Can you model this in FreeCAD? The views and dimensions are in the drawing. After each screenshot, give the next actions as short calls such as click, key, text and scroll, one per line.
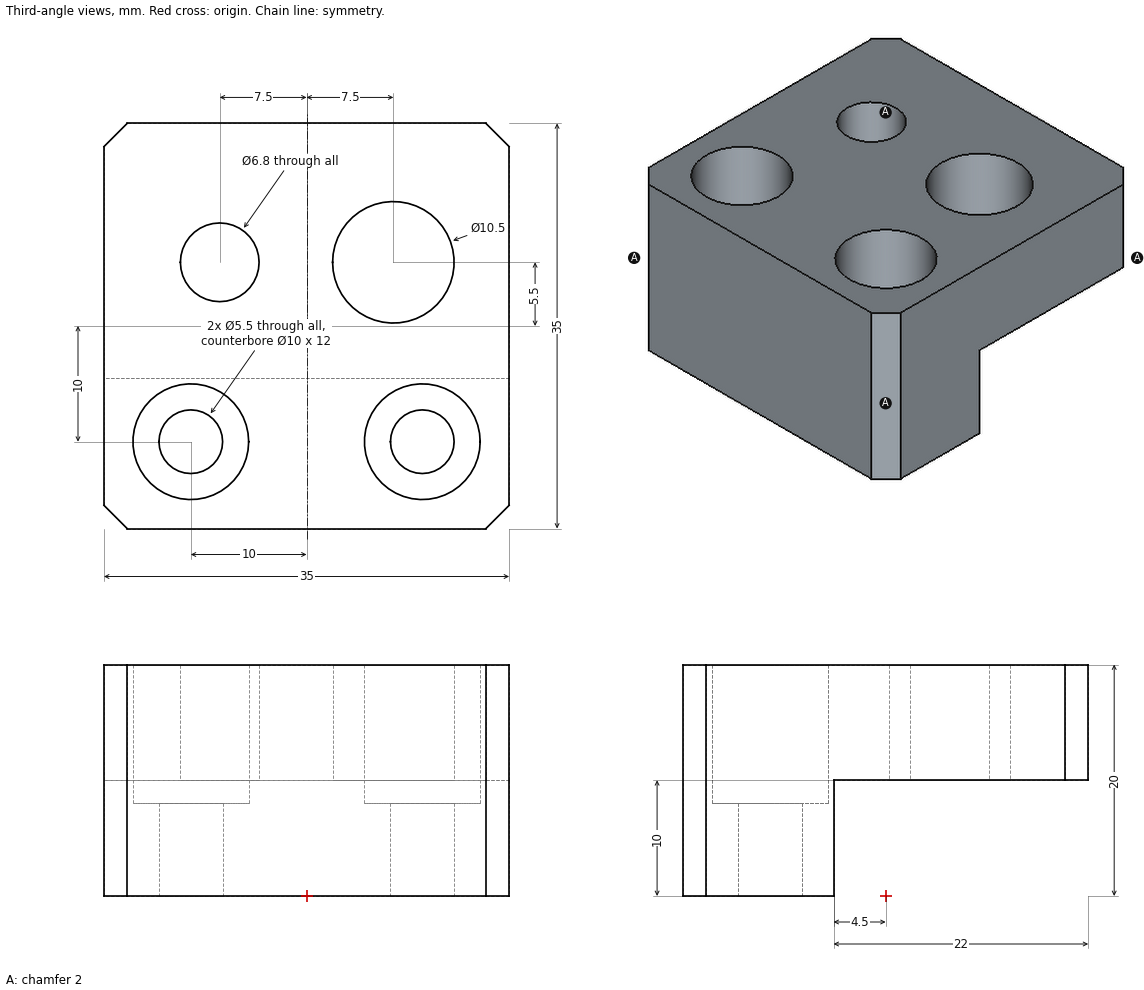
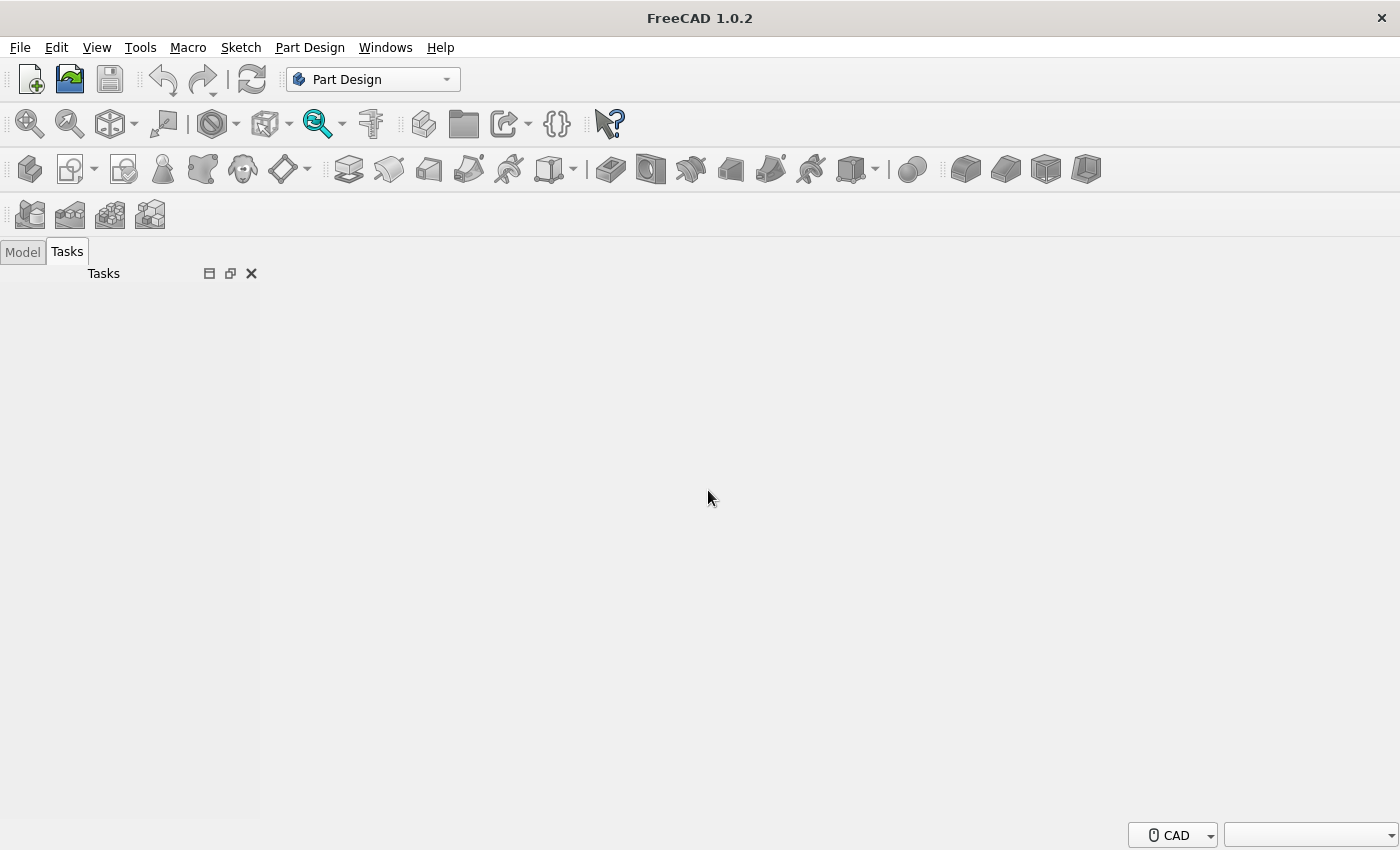
key(ctrl+n)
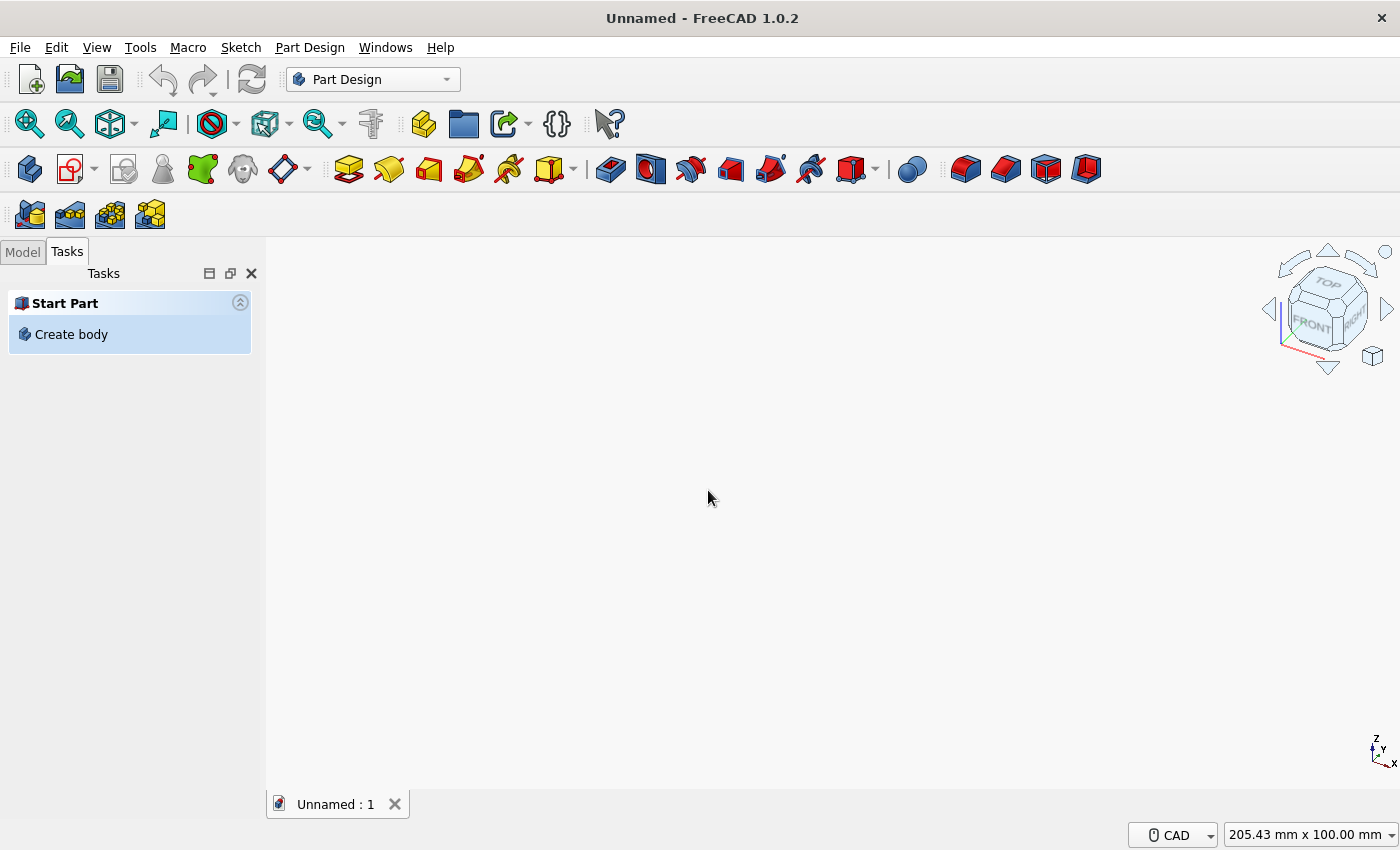
click(70, 170)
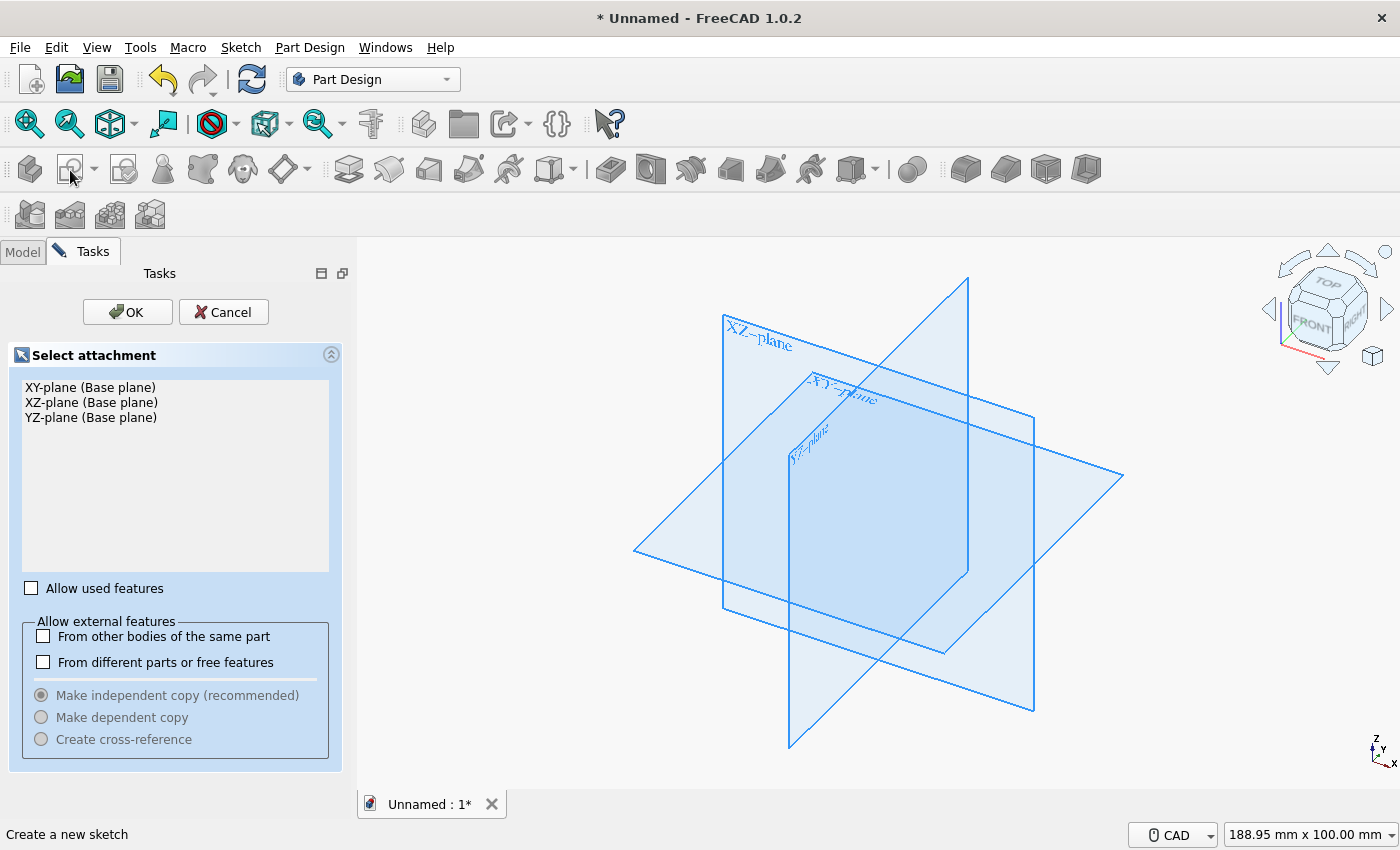
click(82, 388)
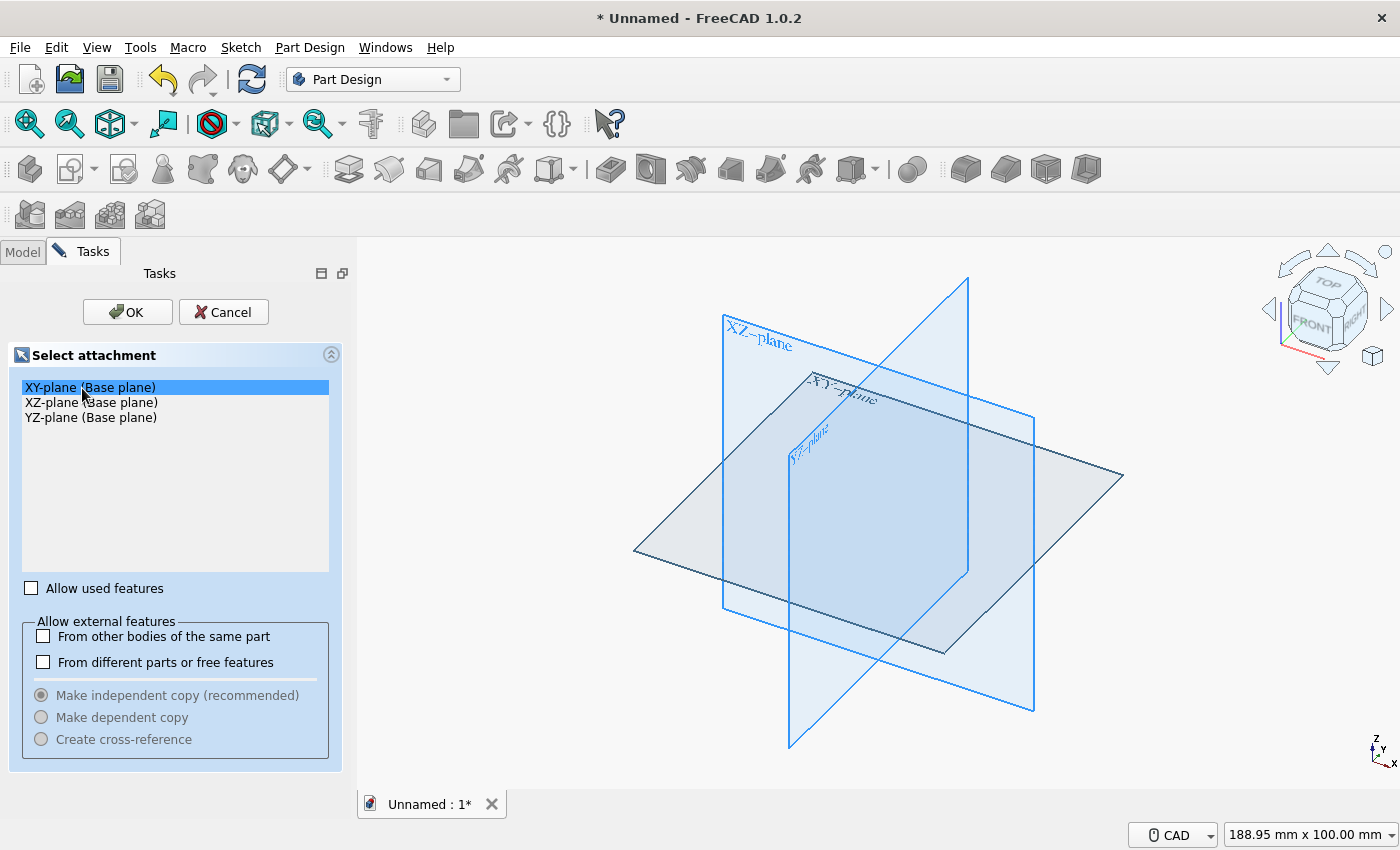
click(128, 312)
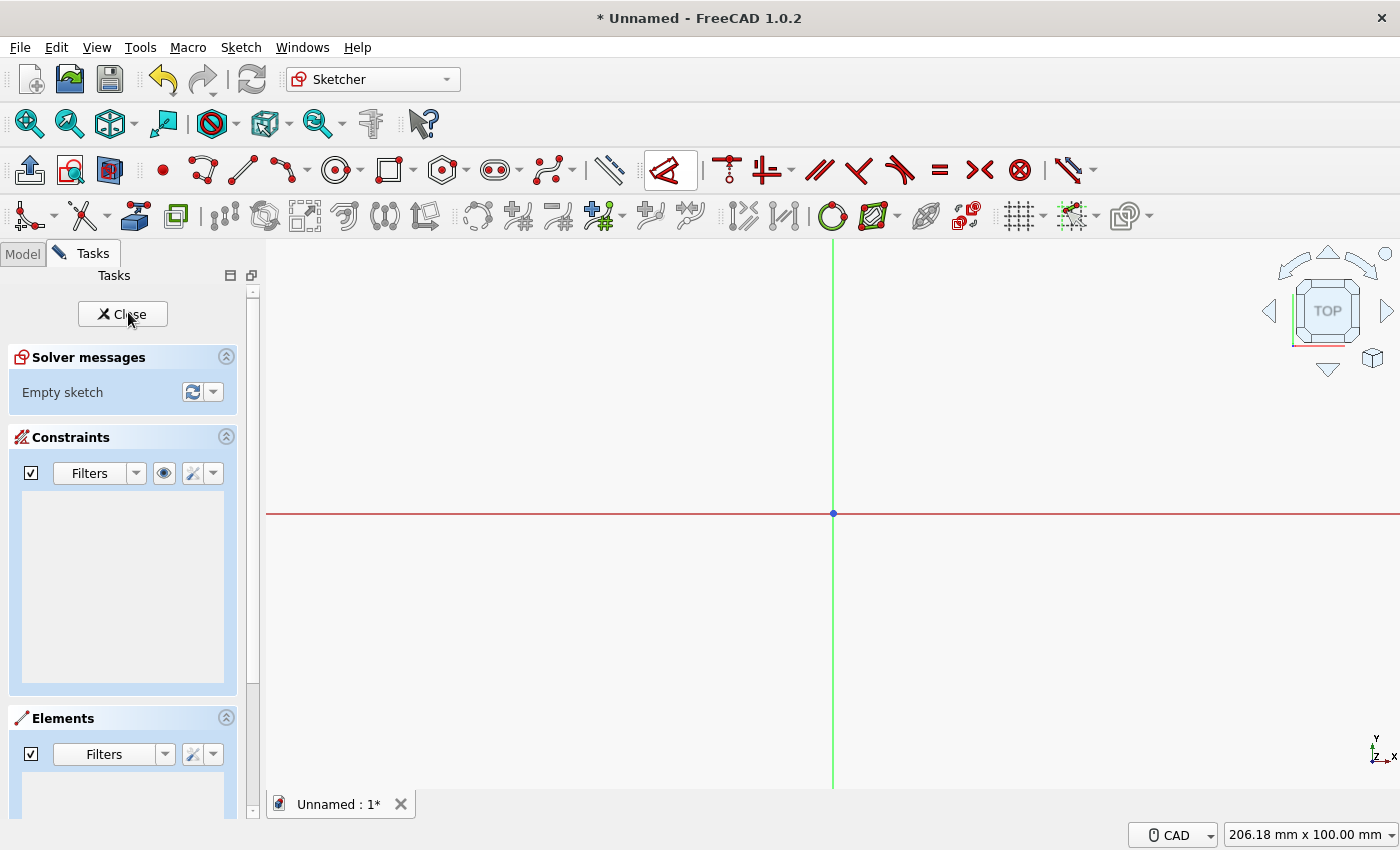
scroll(916, 514, up, 3)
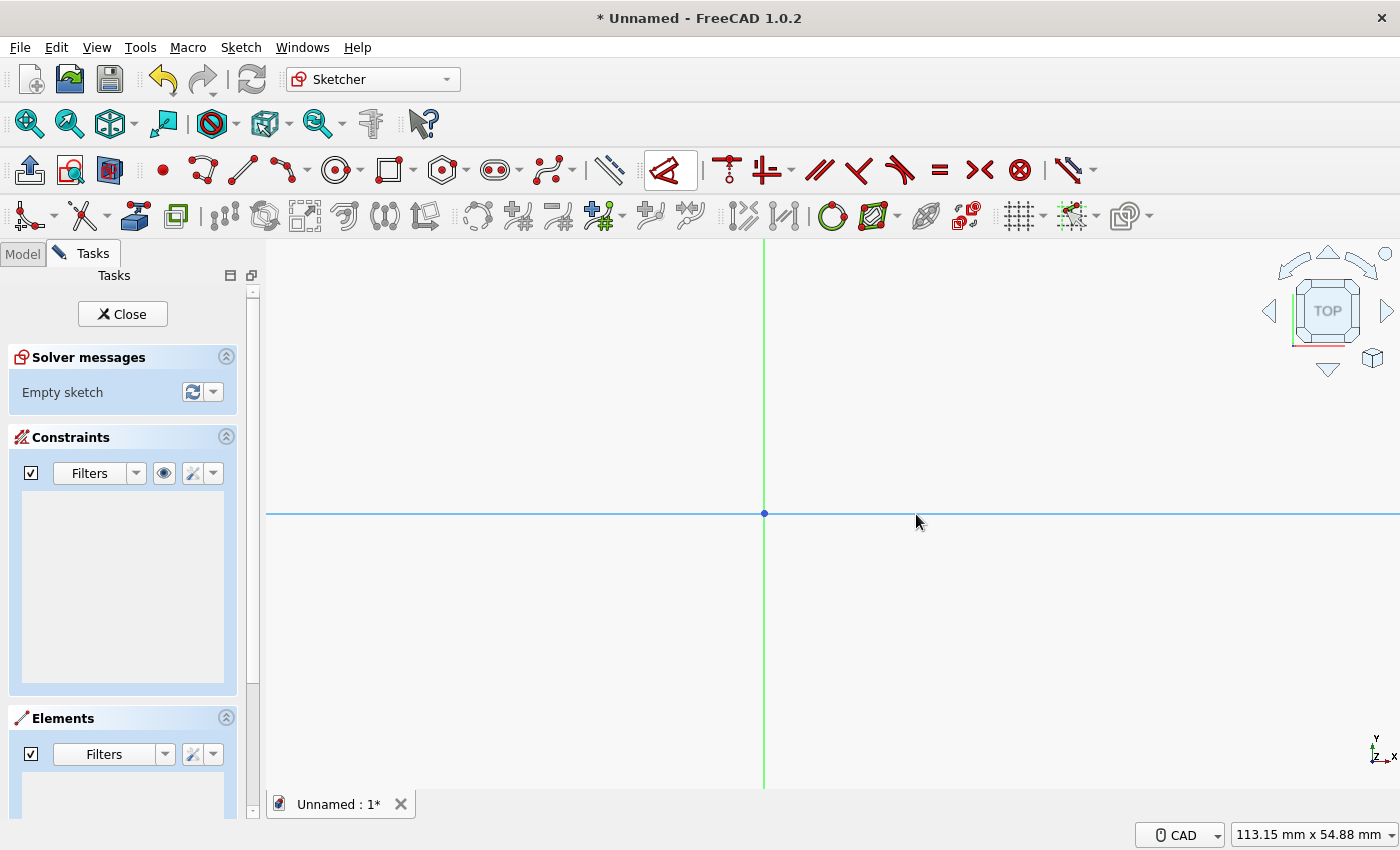
click(416, 170)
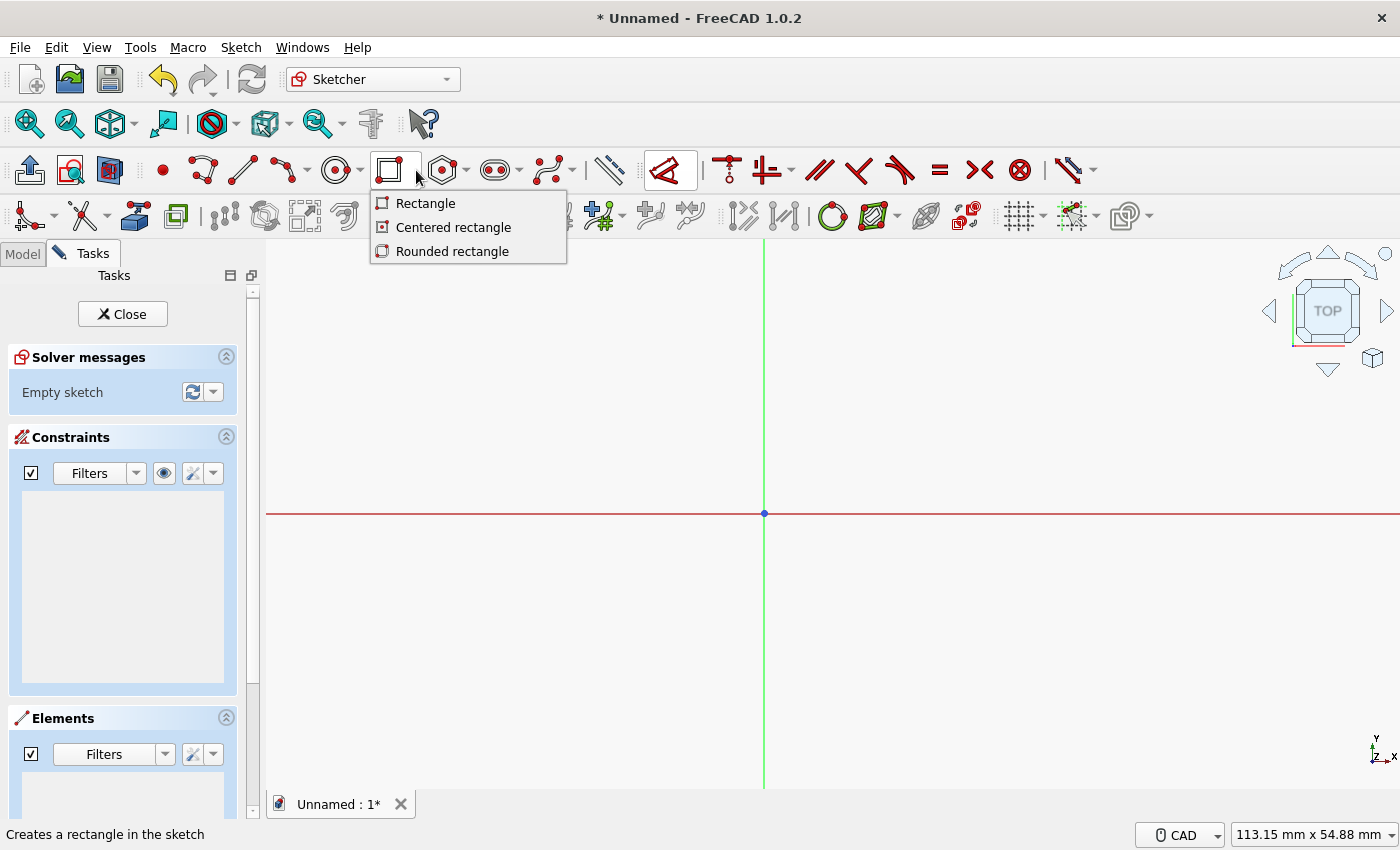
click(468, 227)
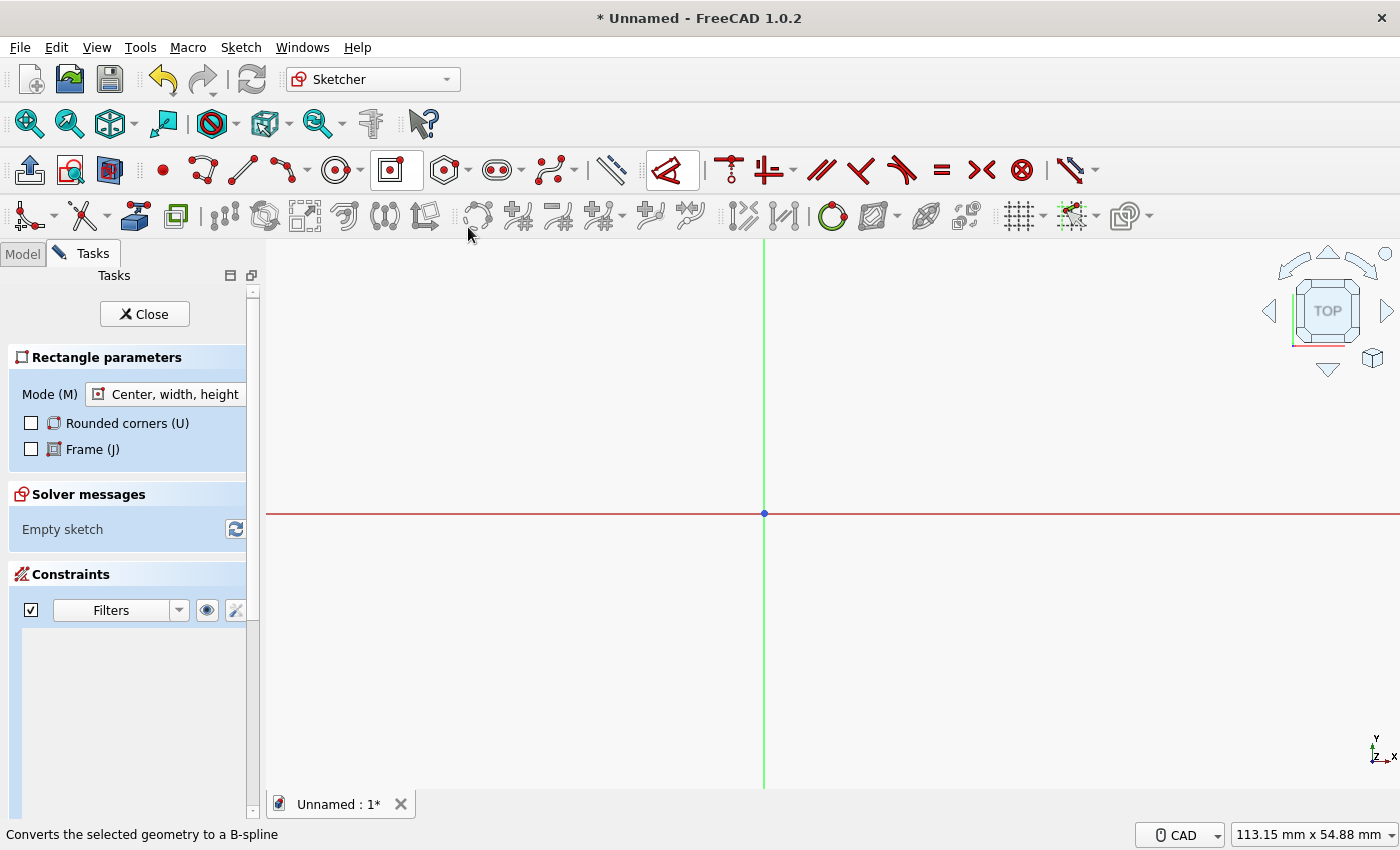
click(764, 514)
move(940, 338)